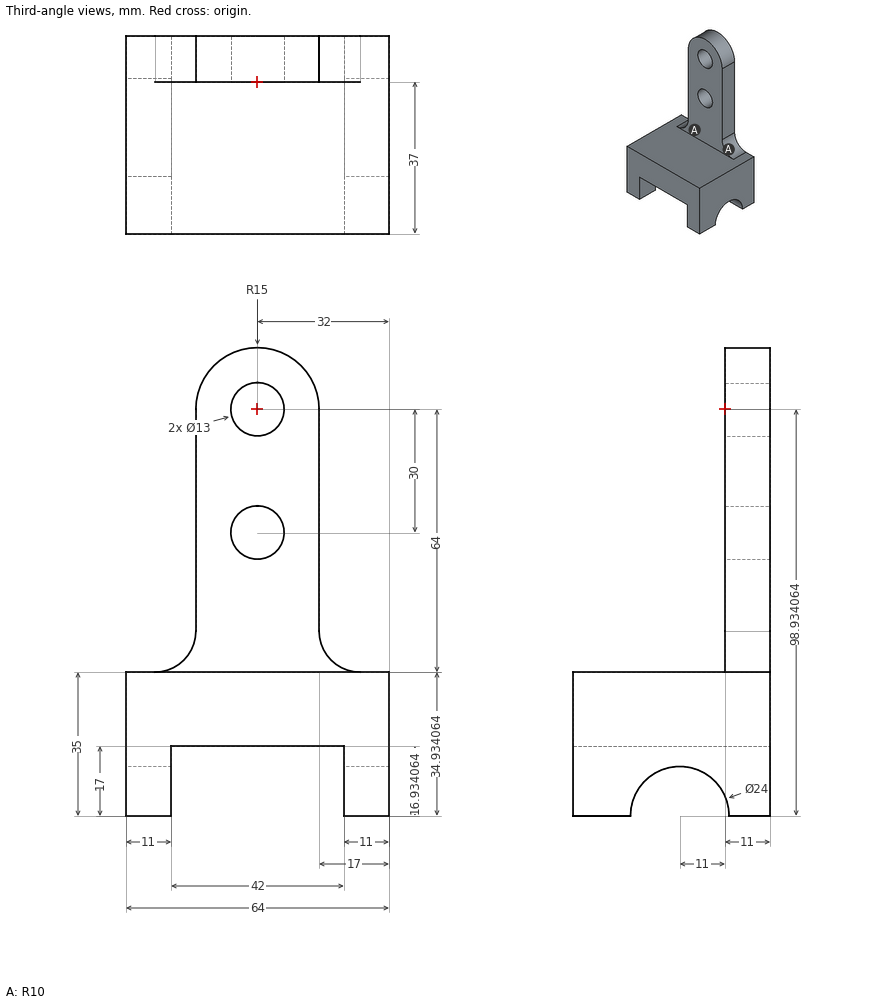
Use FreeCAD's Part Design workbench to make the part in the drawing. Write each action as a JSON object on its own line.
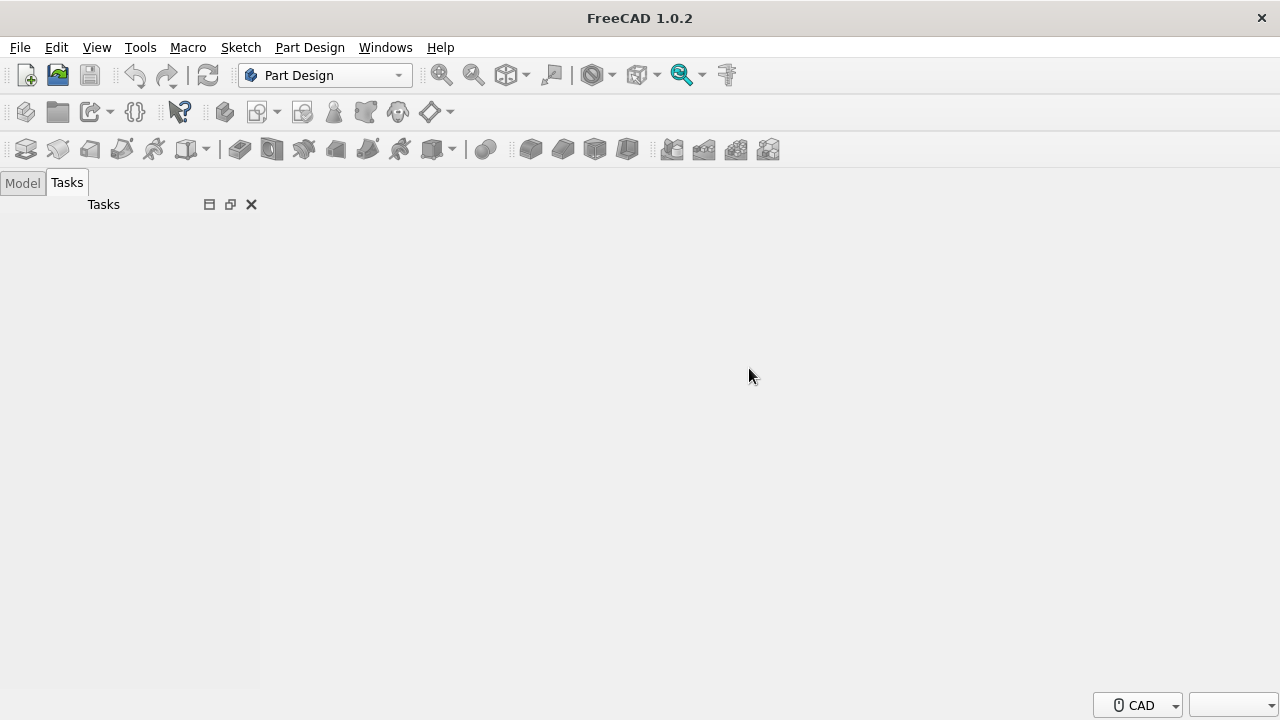
{"action": "left_click", "coordinate": [26, 76]}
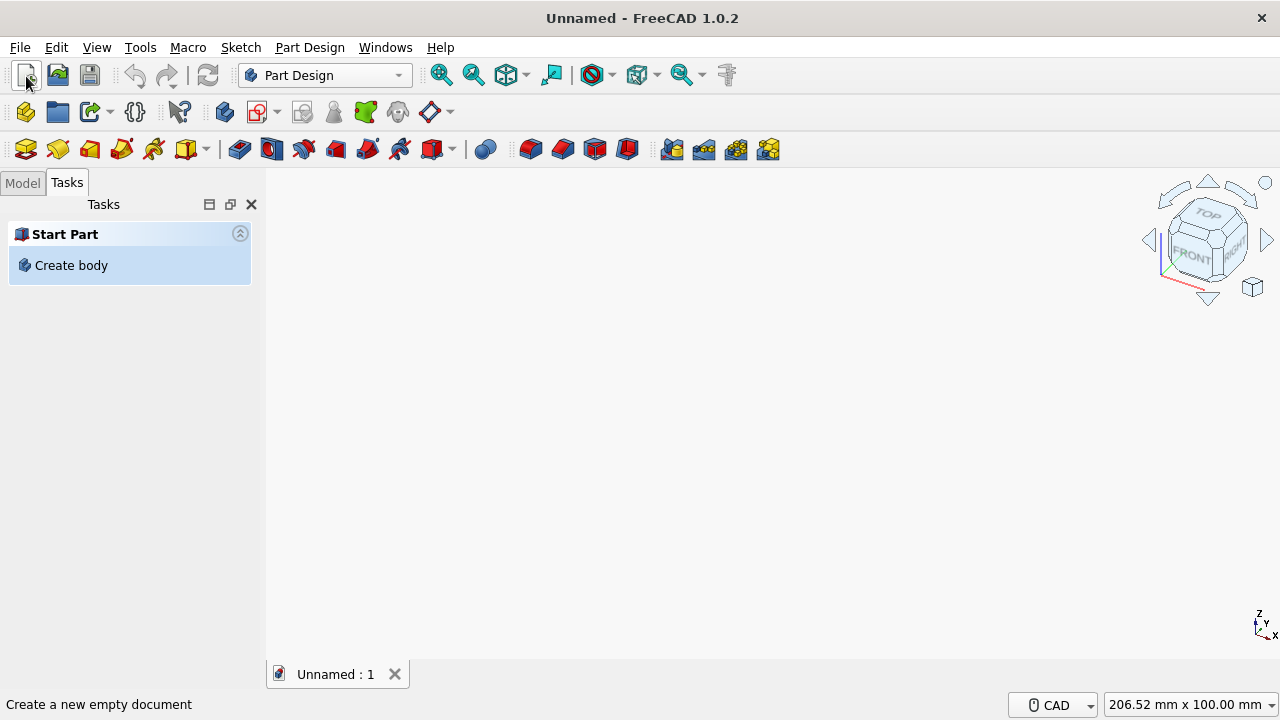
{"action": "left_click", "coordinate": [258, 112]}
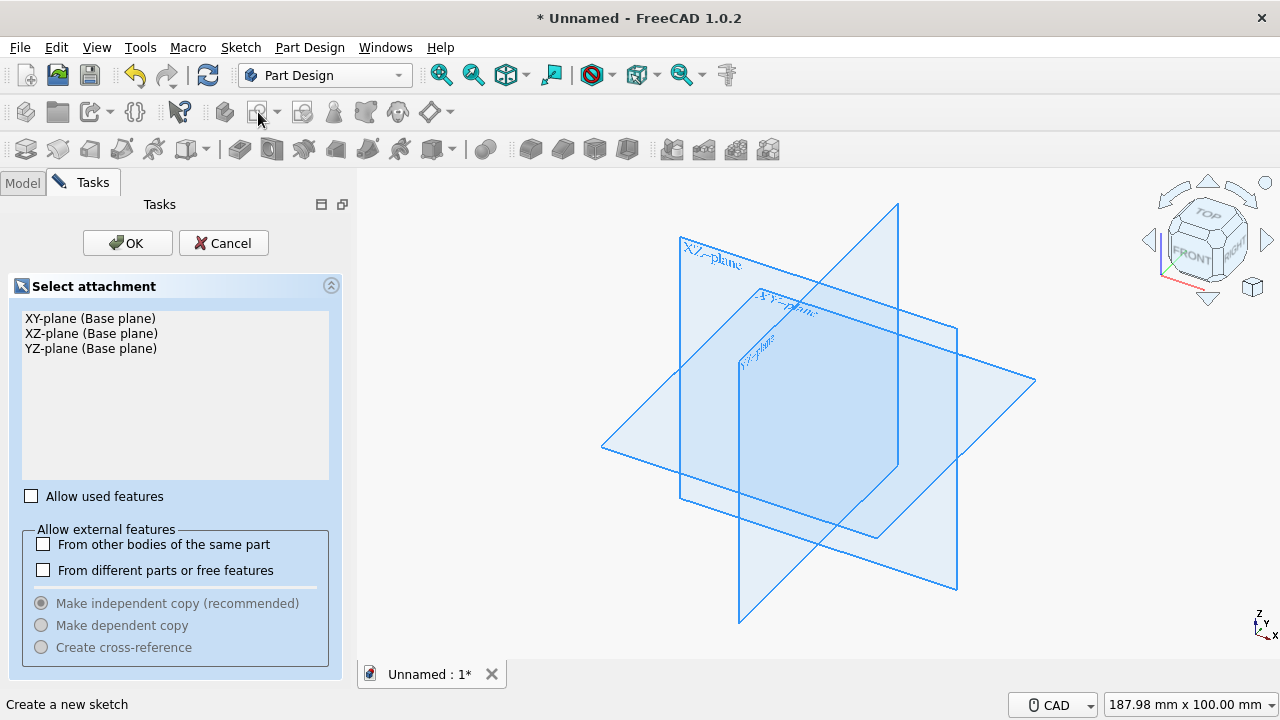
{"action": "left_click", "coordinate": [82, 334]}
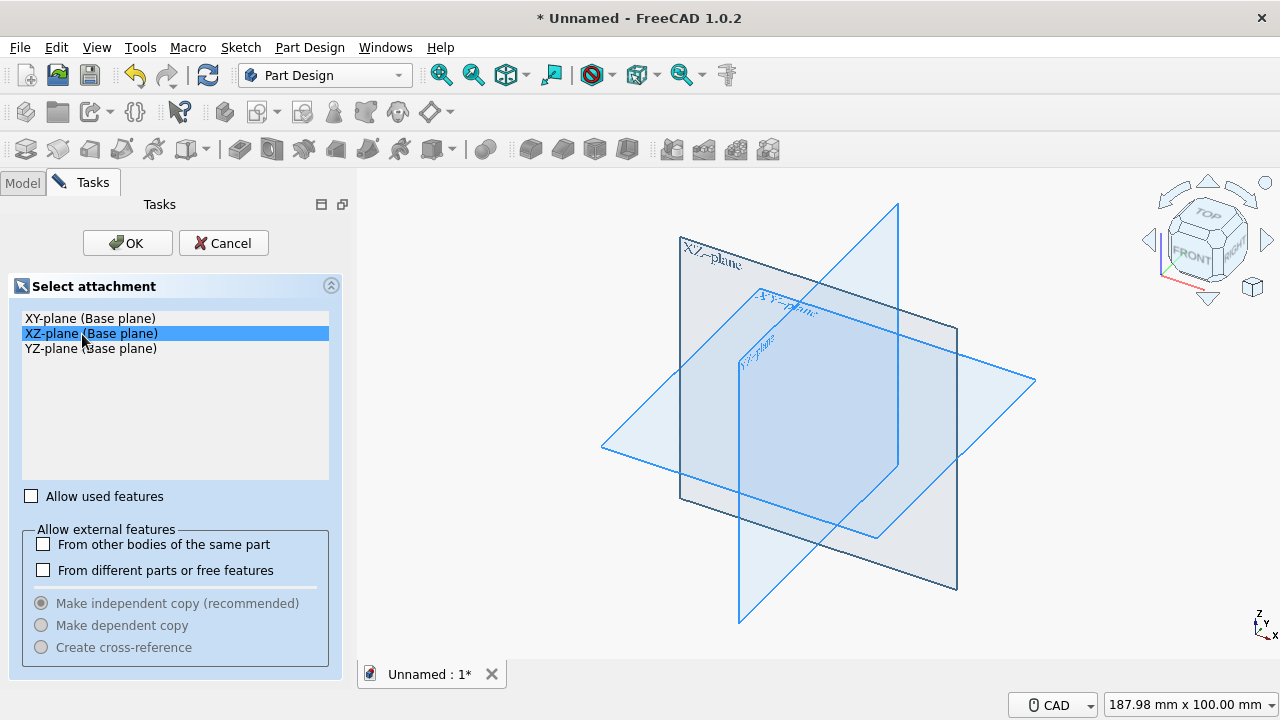
{"action": "left_click", "coordinate": [128, 243]}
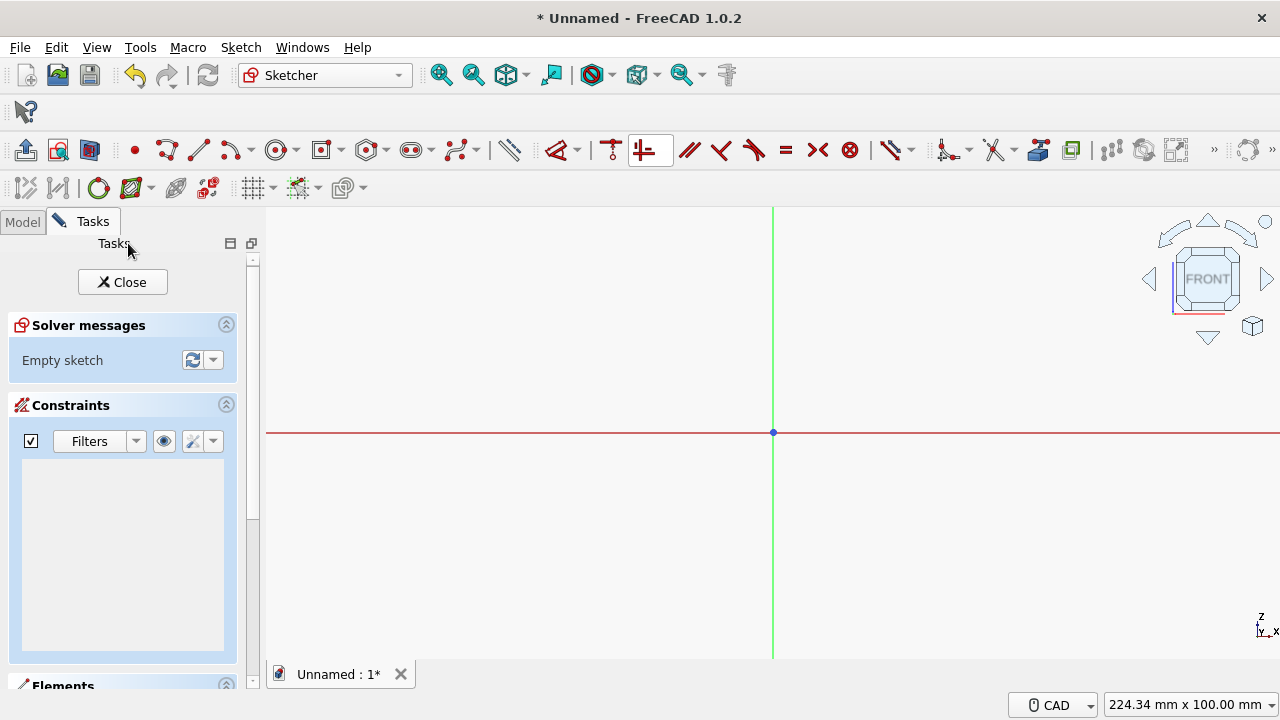
{"action": "scroll", "coordinate": [621, 235], "scroll_direction": "down", "scroll_amount": 3}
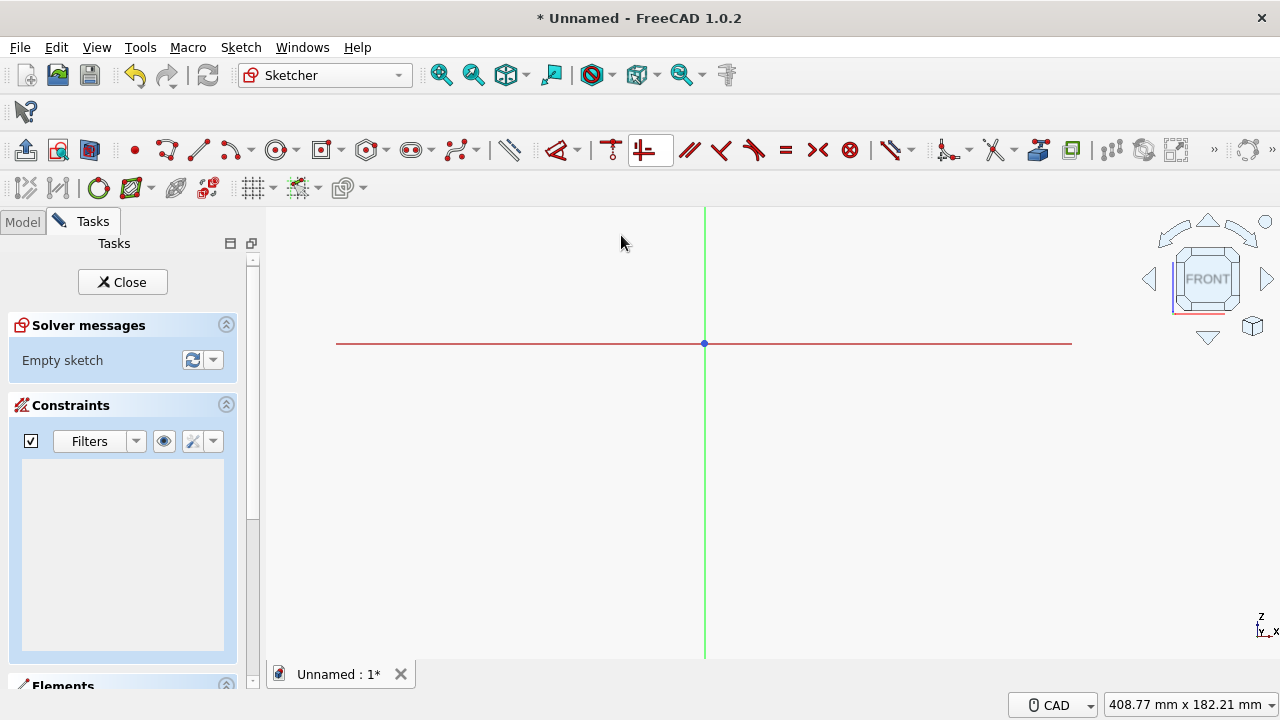
{"action": "left_click", "coordinate": [168, 150]}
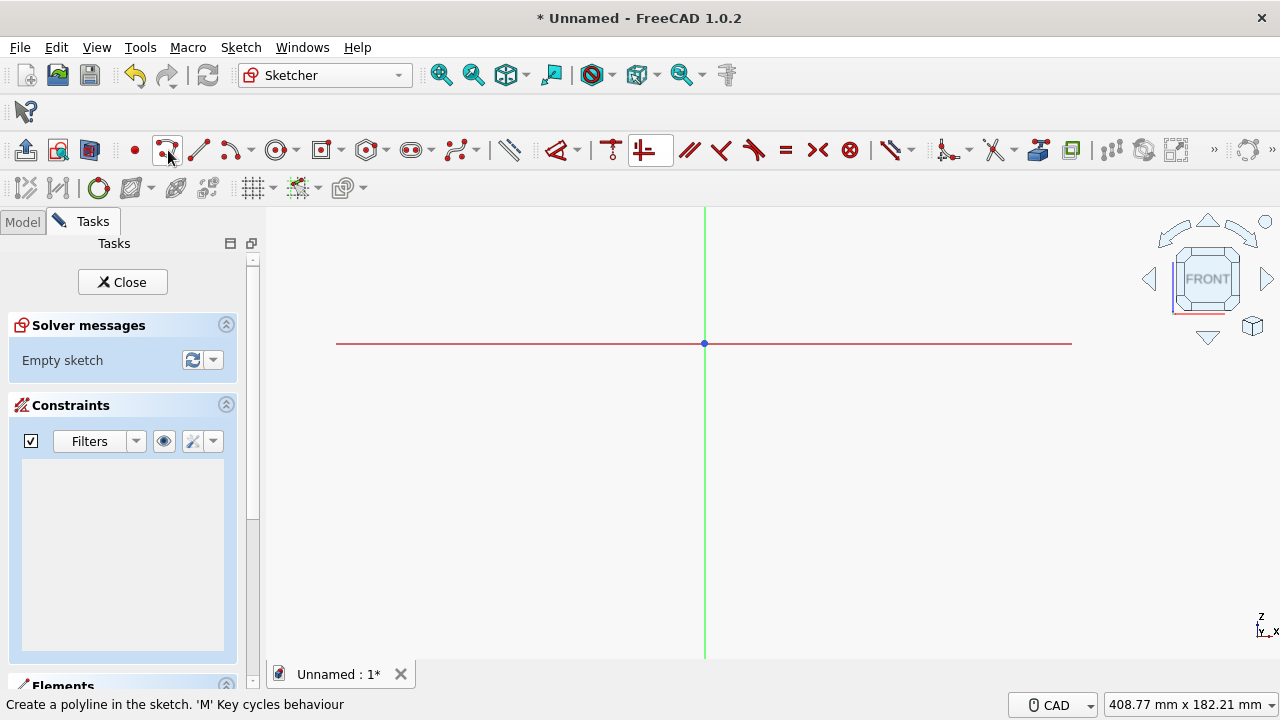
{"action": "left_click", "coordinate": [742, 344]}
{"action": "left_click", "coordinate": [742, 502]}
{"action": "left_click", "coordinate": [784, 502]}
{"action": "left_click", "coordinate": [784, 589]}
{"action": "left_click", "coordinate": [757, 589]}
{"action": "left_click", "coordinate": [757, 547]}
{"action": "left_click", "coordinate": [652, 547]}
{"action": "left_click", "coordinate": [652, 589]}
{"action": "left_click", "coordinate": [625, 589]}
{"action": "left_click", "coordinate": [625, 502]}
{"action": "left_click", "coordinate": [667, 502]}
{"action": "left_click", "coordinate": [667, 344]}
{"action": "right_click", "coordinate": [667, 344]}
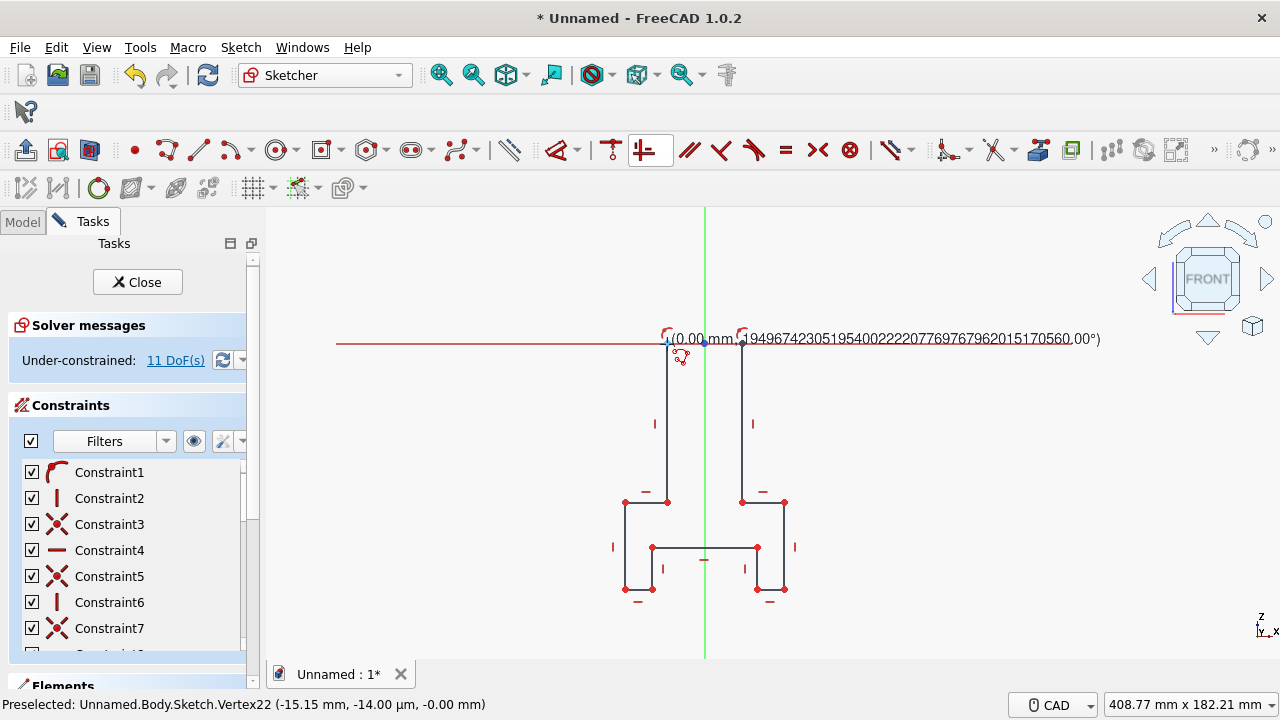
{"action": "key", "text": "g 3 a"}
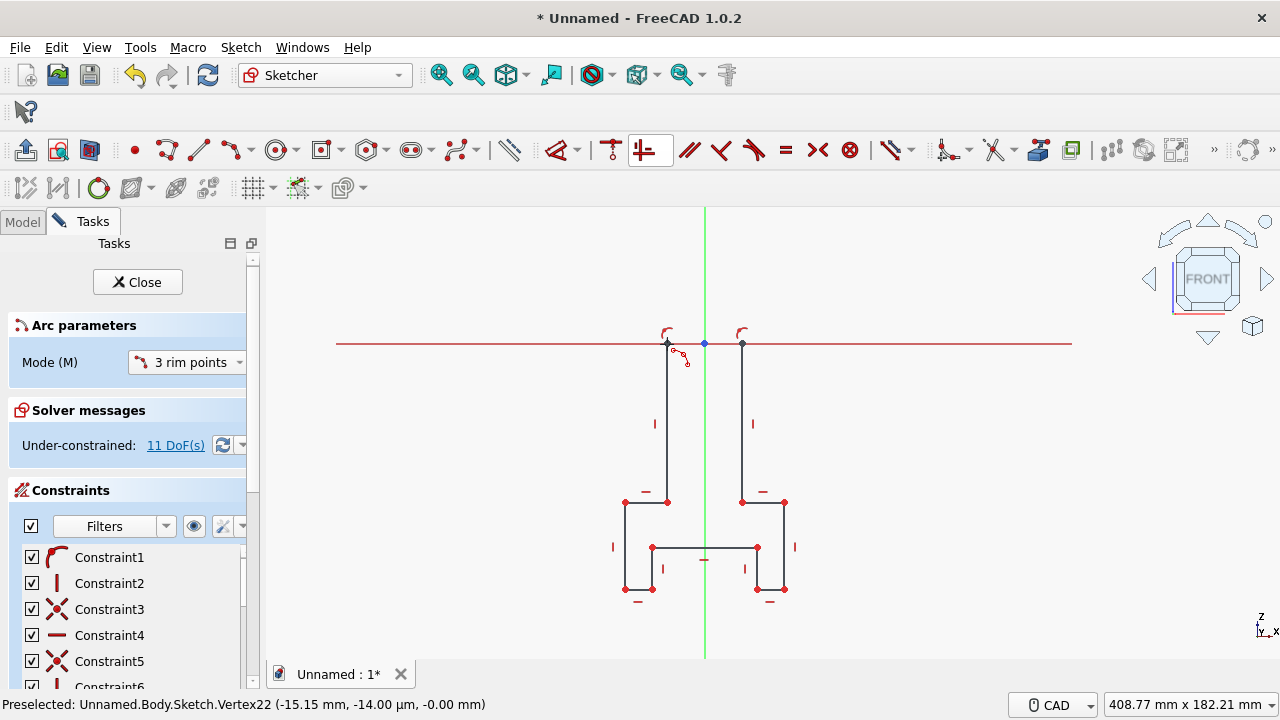
{"action": "left_click", "coordinate": [667, 344]}
{"action": "left_click", "coordinate": [742, 344]}
{"action": "left_click", "coordinate": [726, 314]}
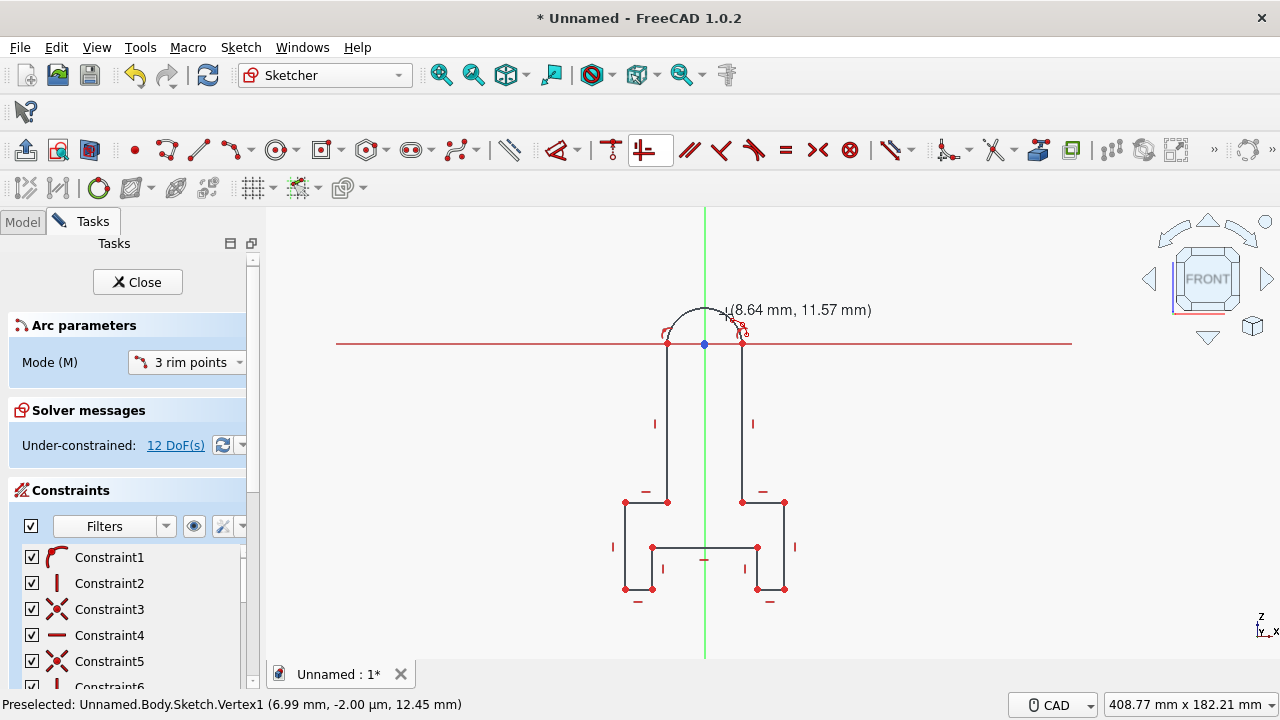
{"action": "left_click", "coordinate": [276, 150]}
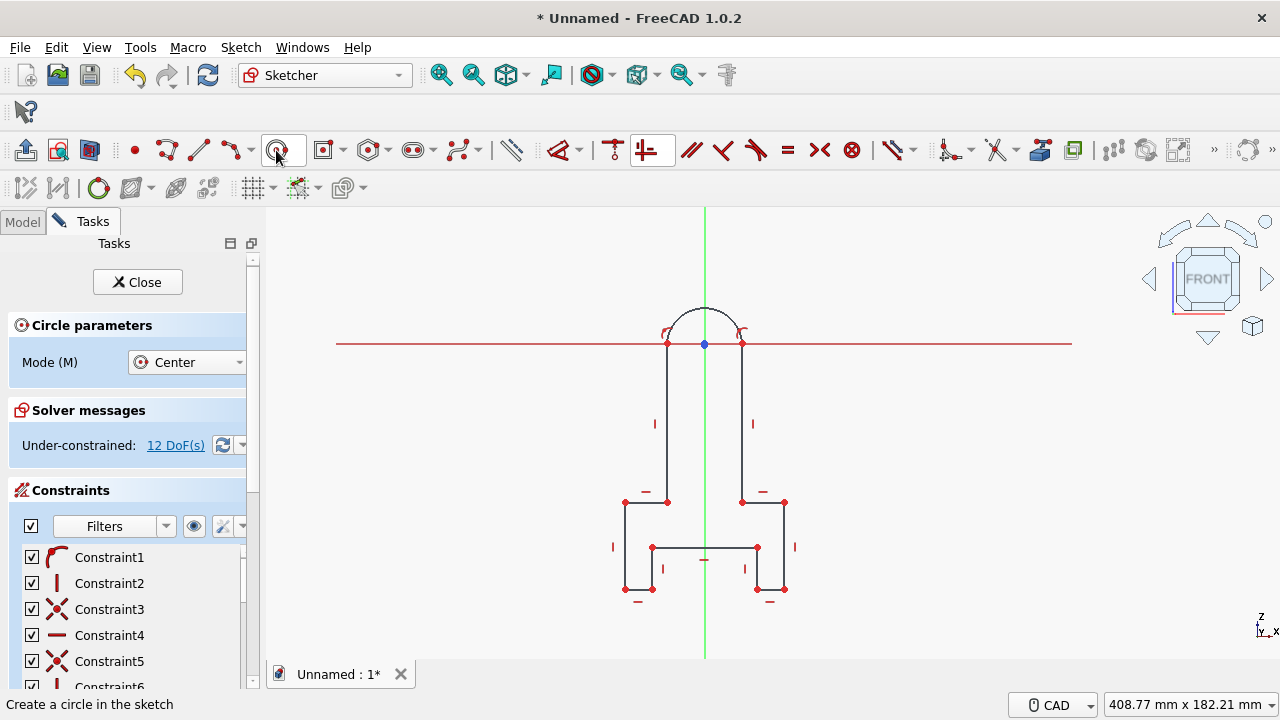
{"action": "scroll", "coordinate": [705, 344], "scroll_direction": "up", "scroll_amount": 2}